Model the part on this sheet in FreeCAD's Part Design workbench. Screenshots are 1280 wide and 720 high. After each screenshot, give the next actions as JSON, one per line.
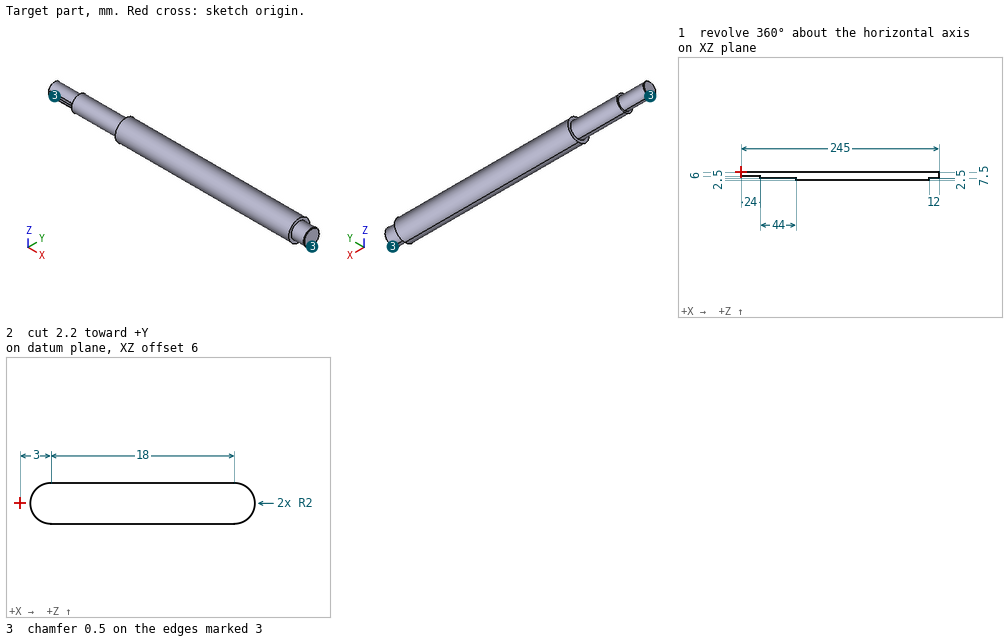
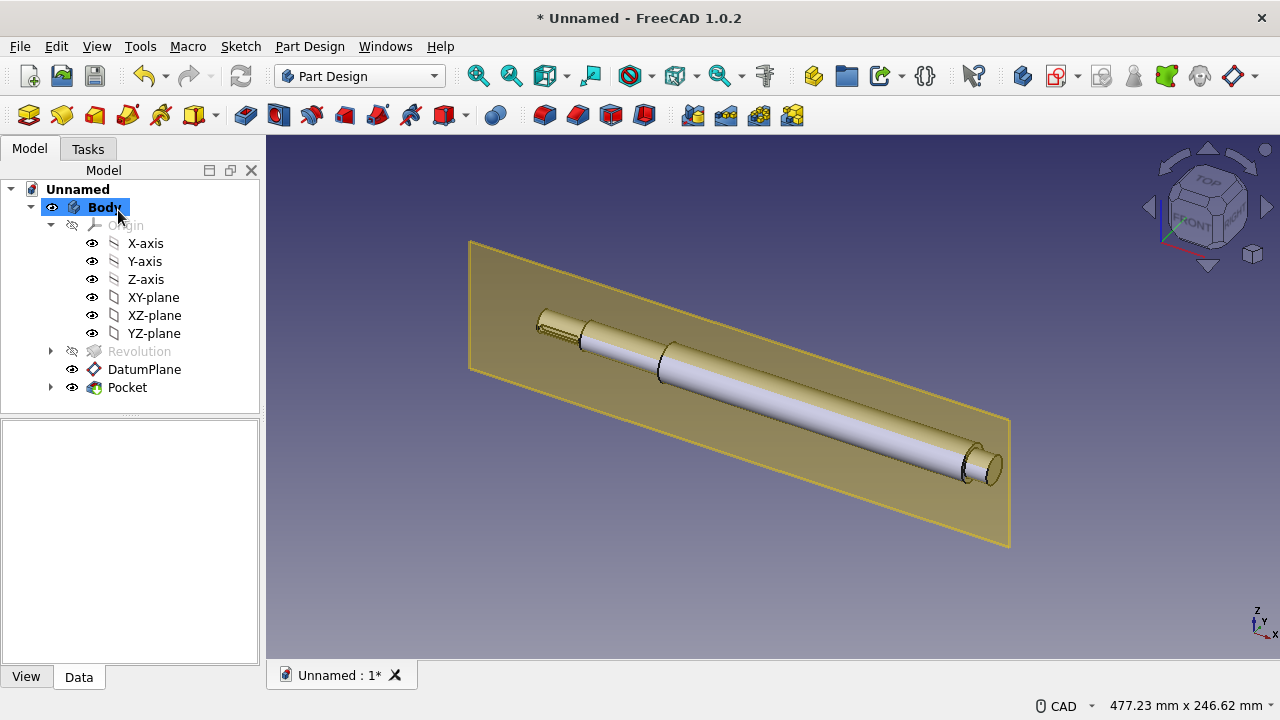
{"action": "left_click", "coordinate": [117, 369]}
{"action": "key", "text": "space"}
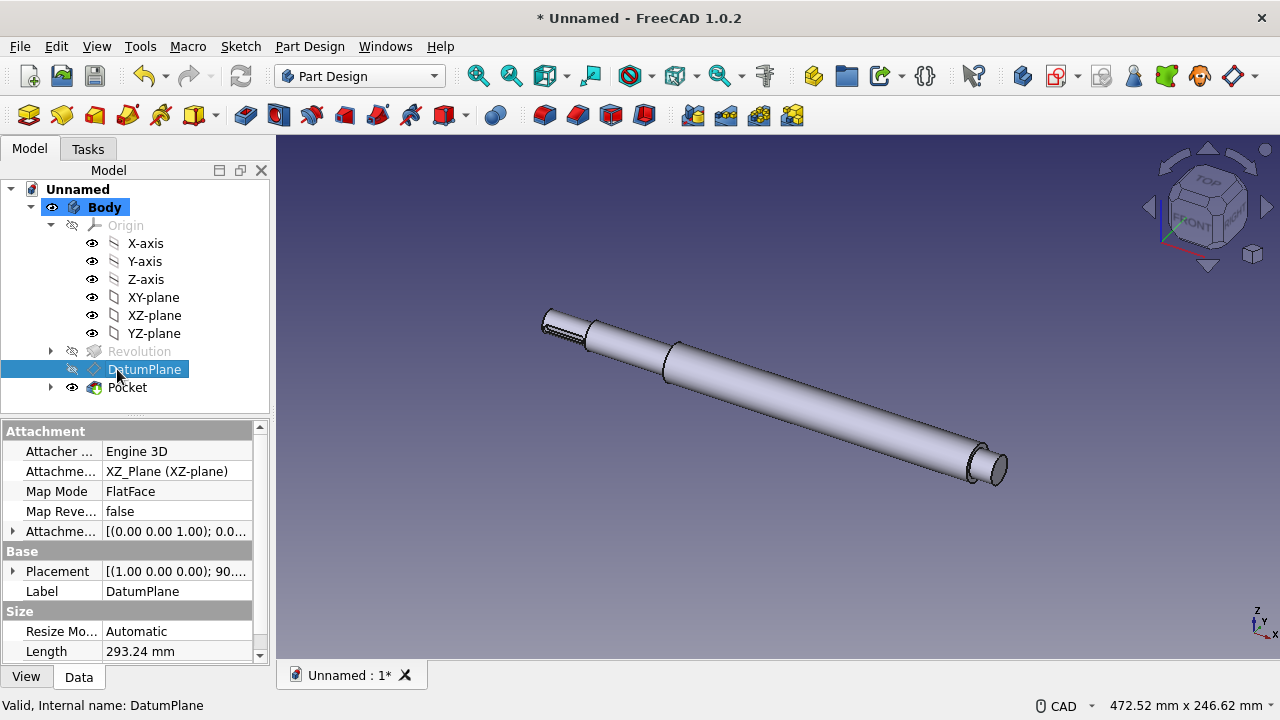
{"action": "left_click", "coordinate": [549, 310]}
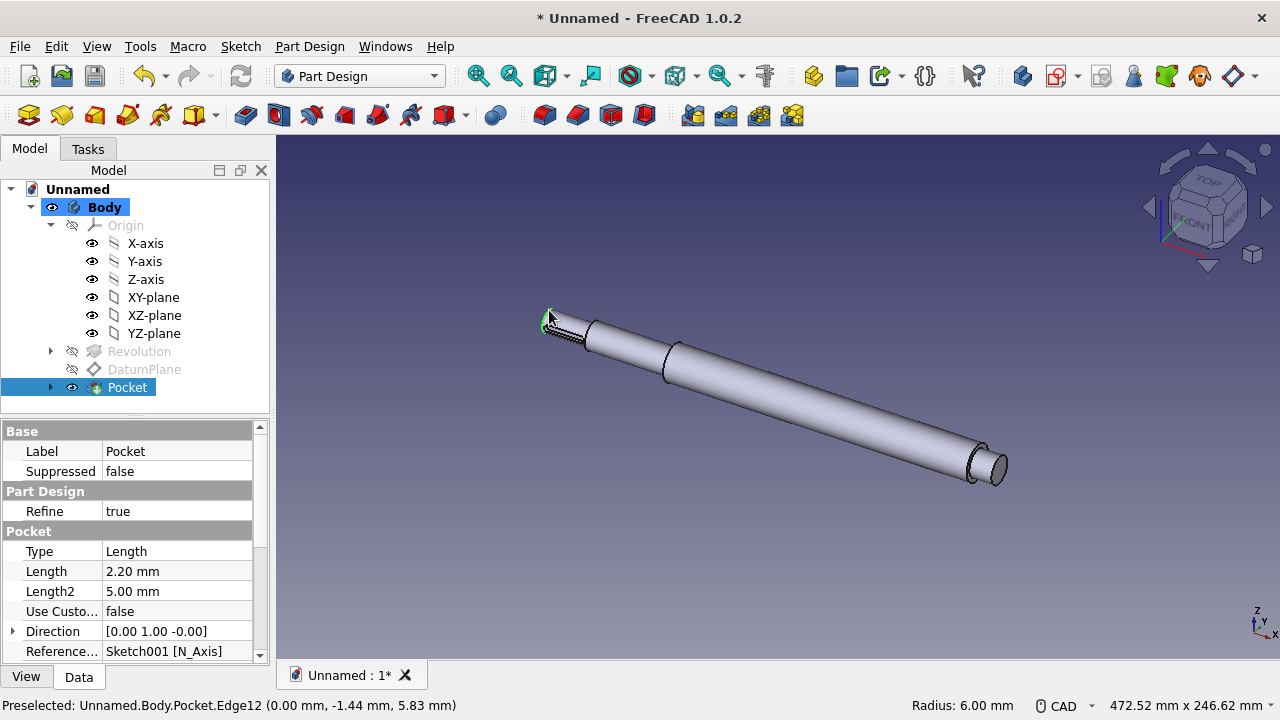
{"action": "left_click", "coordinate": [999, 456], "text": "ctrl"}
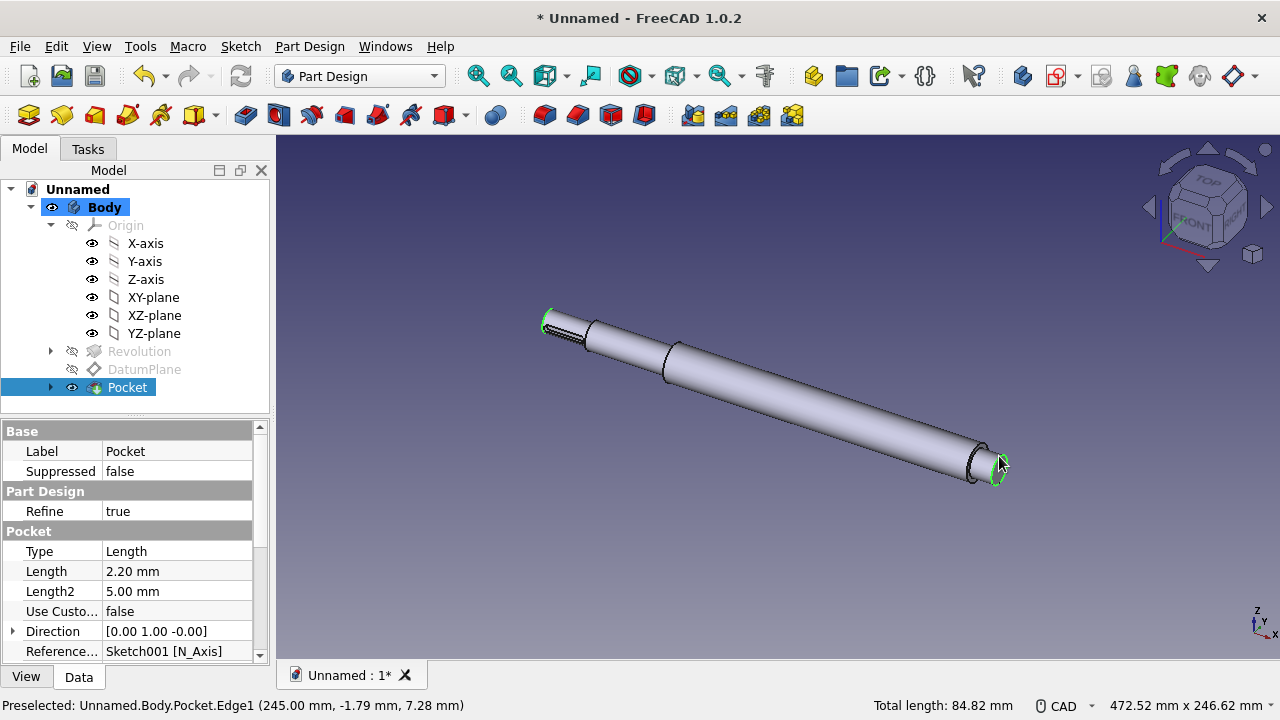
{"action": "left_click", "coordinate": [578, 116]}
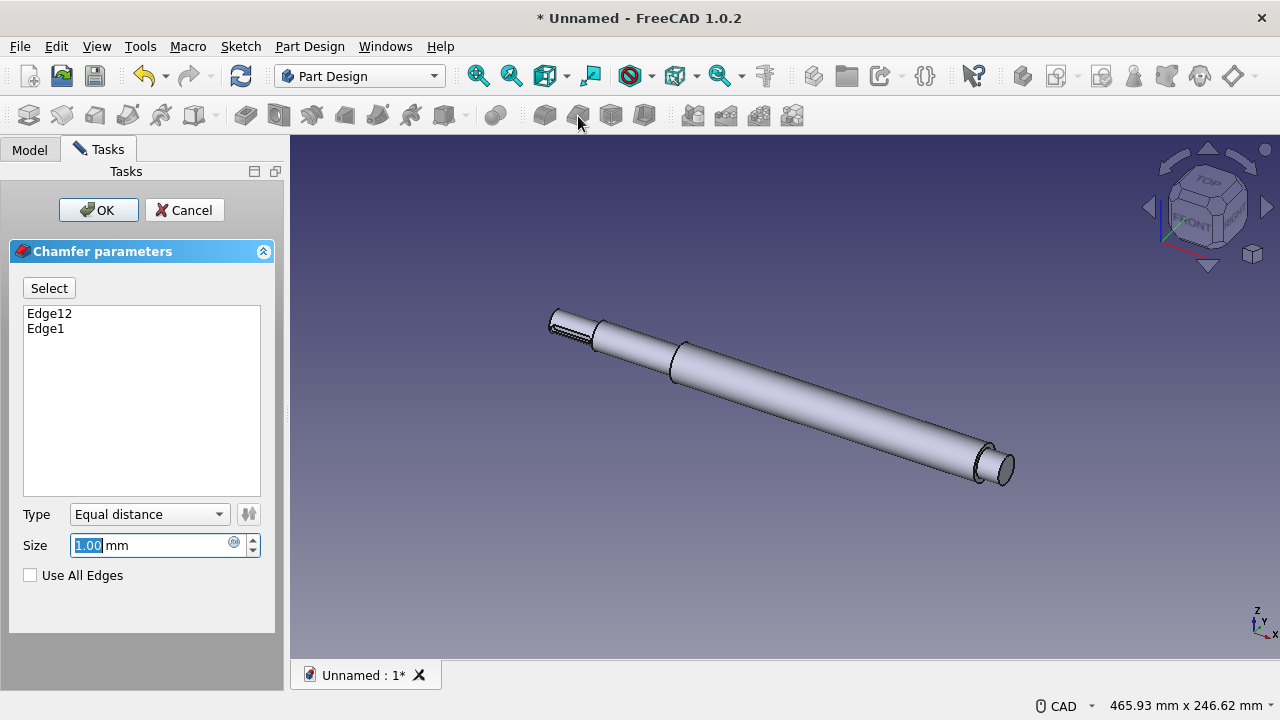
{"action": "type", "text": "0.5"}
{"action": "key", "text": "Tab"}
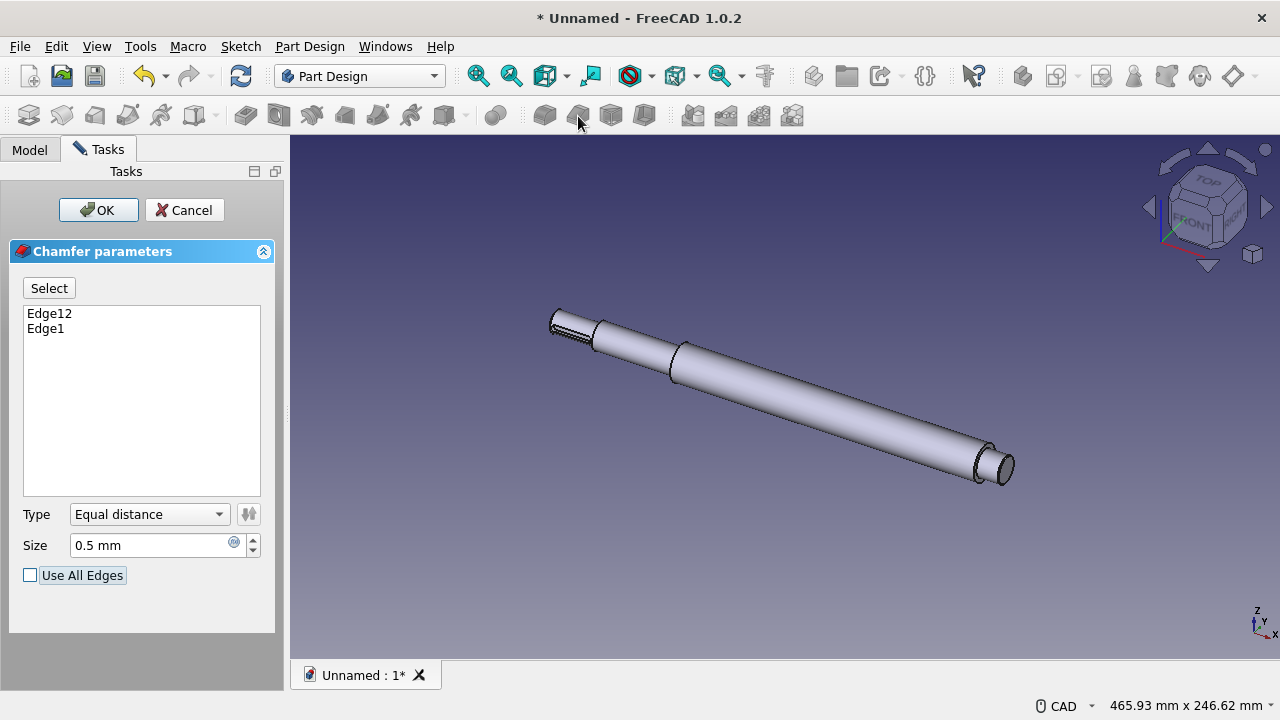
{"action": "left_click", "coordinate": [99, 210]}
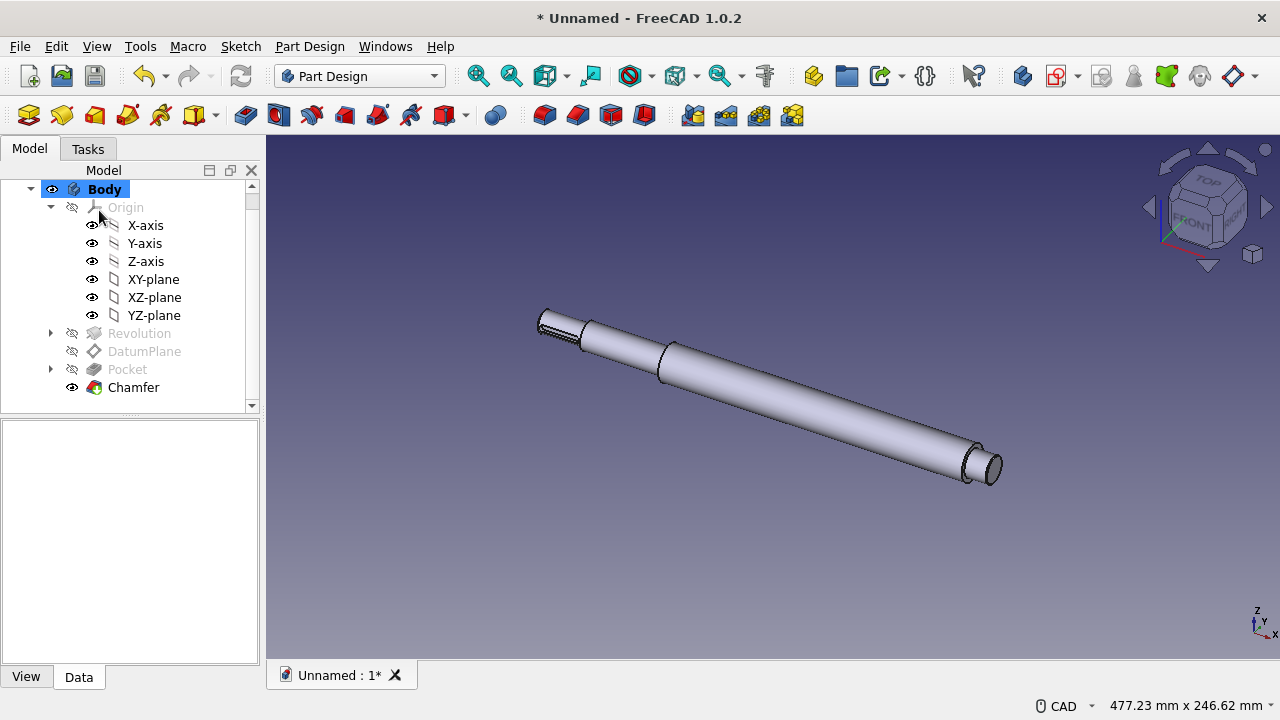
{"action": "key", "text": "0"}